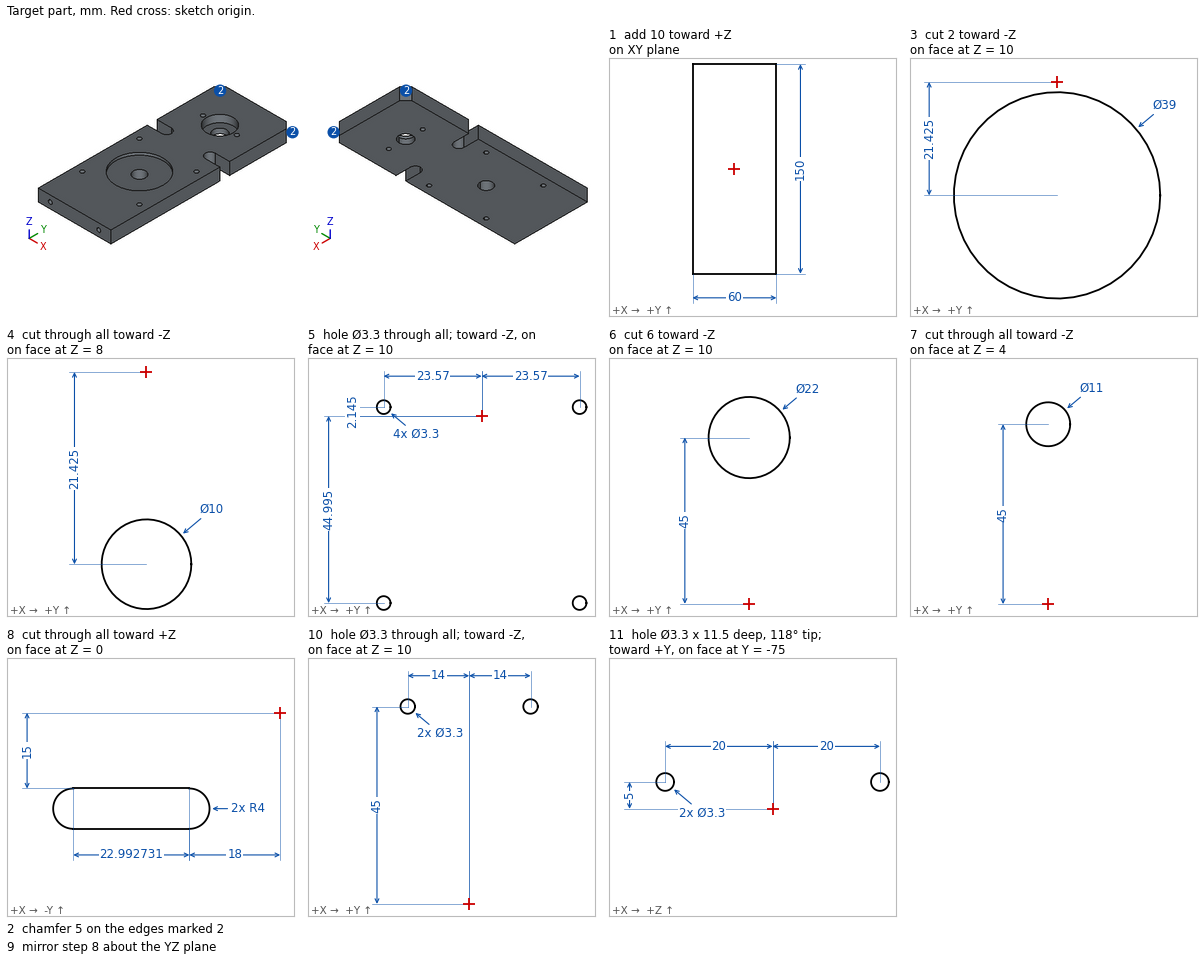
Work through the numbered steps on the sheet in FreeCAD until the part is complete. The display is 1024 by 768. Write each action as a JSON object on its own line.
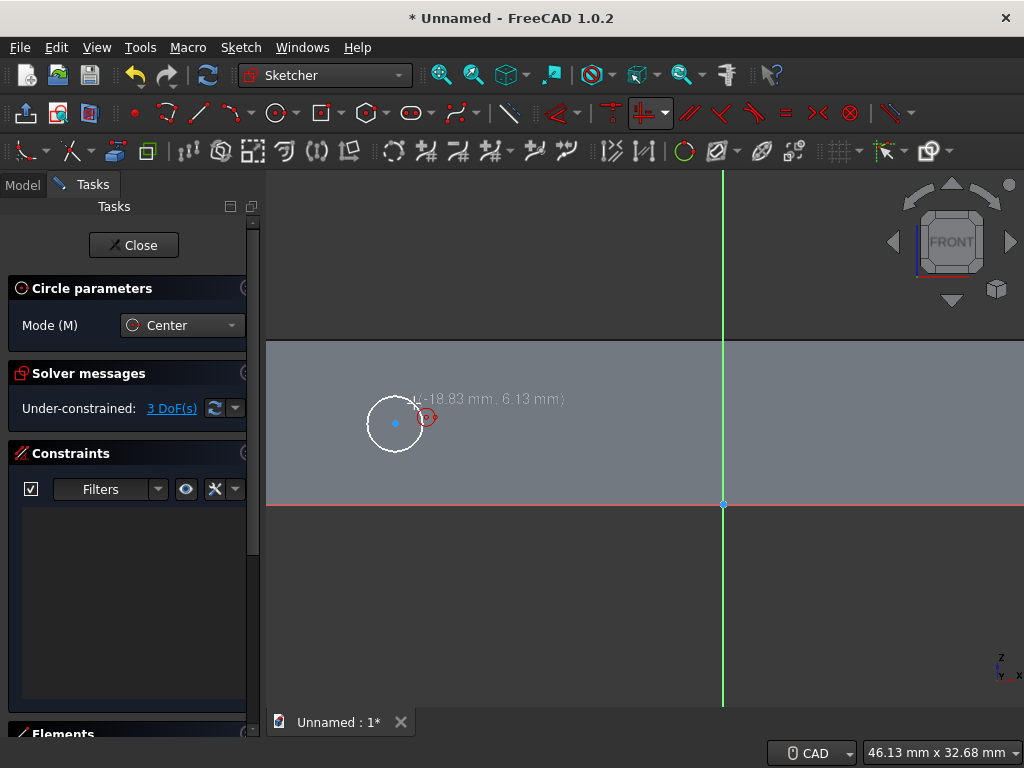
{"action": "scroll", "coordinate": [398, 424], "scroll_direction": "down", "scroll_amount": 3}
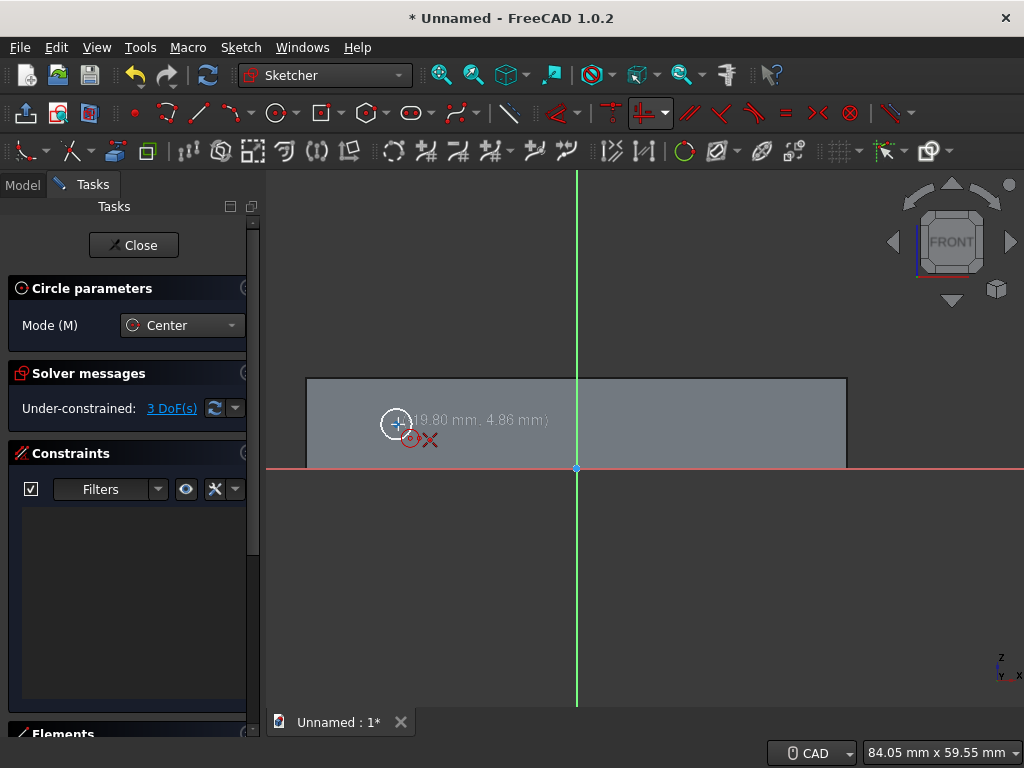
{"action": "scroll", "coordinate": [757, 423], "scroll_direction": "up", "scroll_amount": 3}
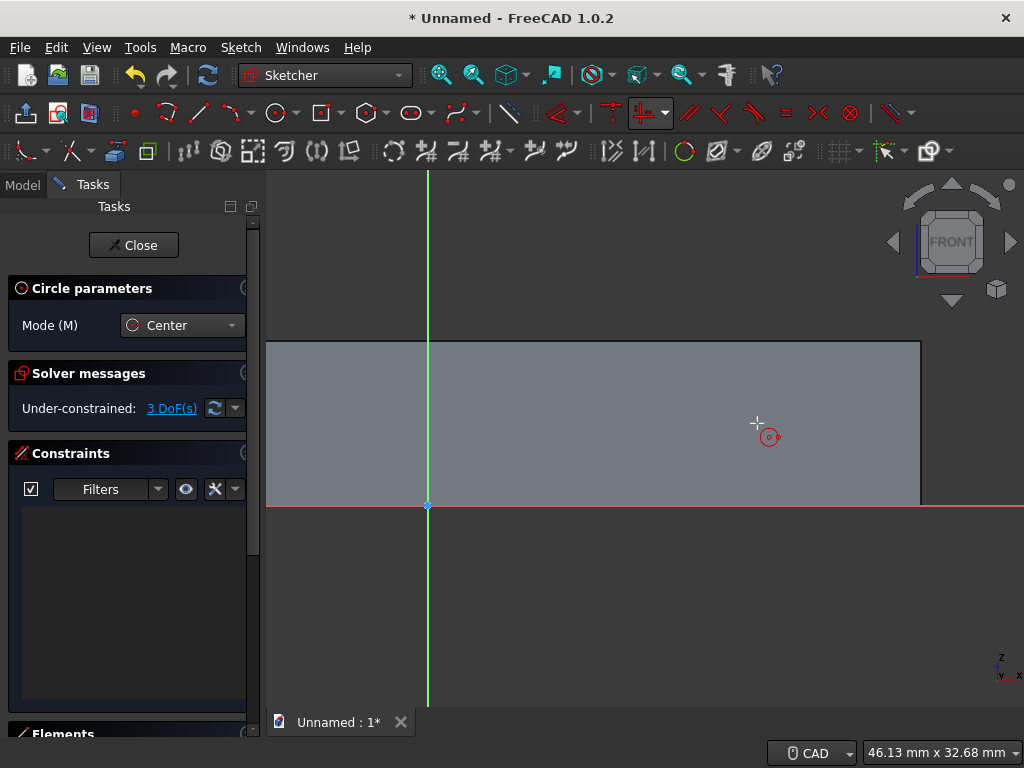
{"action": "left_click", "coordinate": [757, 423]}
{"action": "left_click", "coordinate": [776, 404]}
{"action": "key", "text": "Escape"}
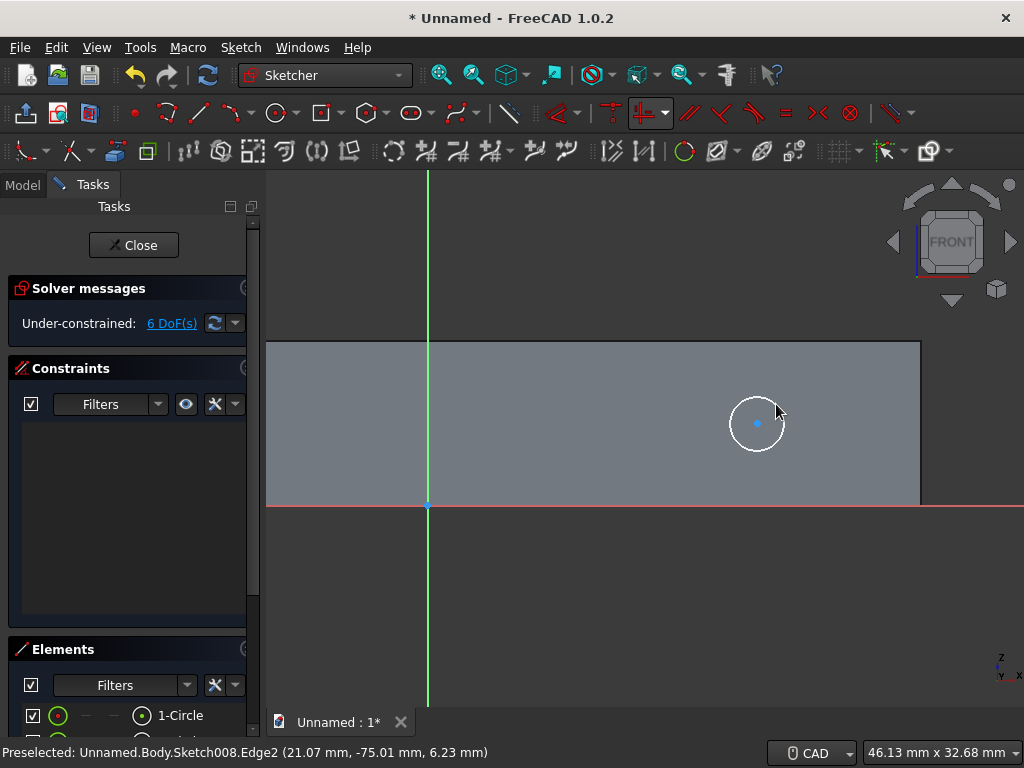
{"action": "scroll", "coordinate": [757, 423], "scroll_direction": "down", "scroll_amount": 3}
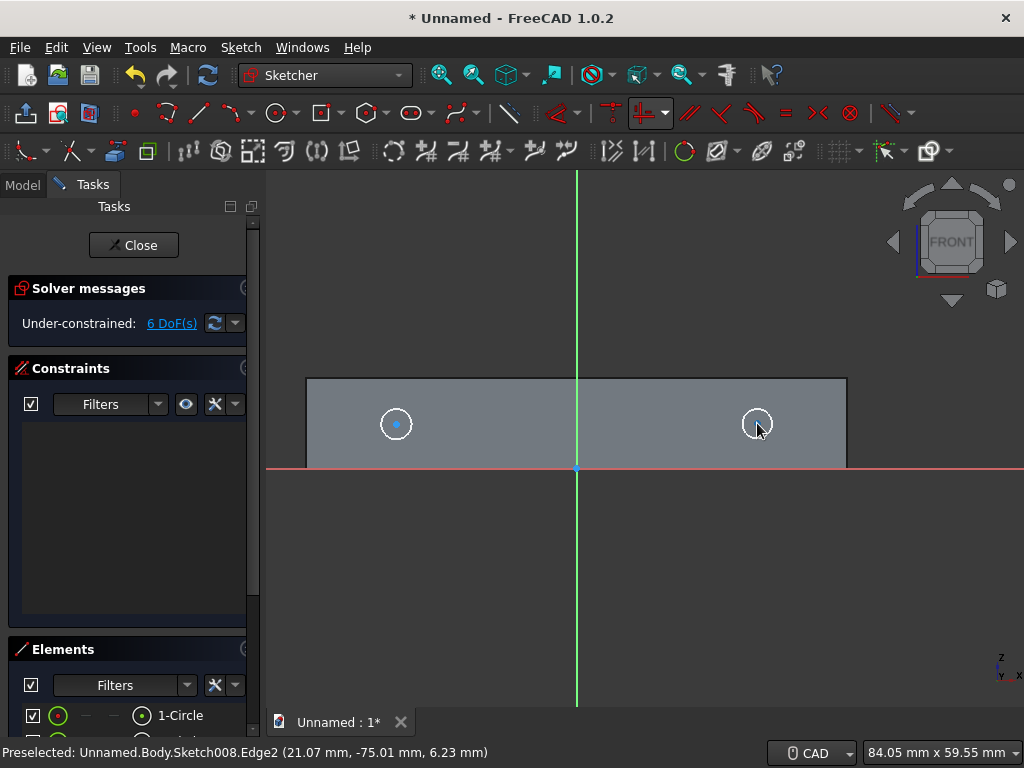
{"action": "left_click", "coordinate": [407, 413]}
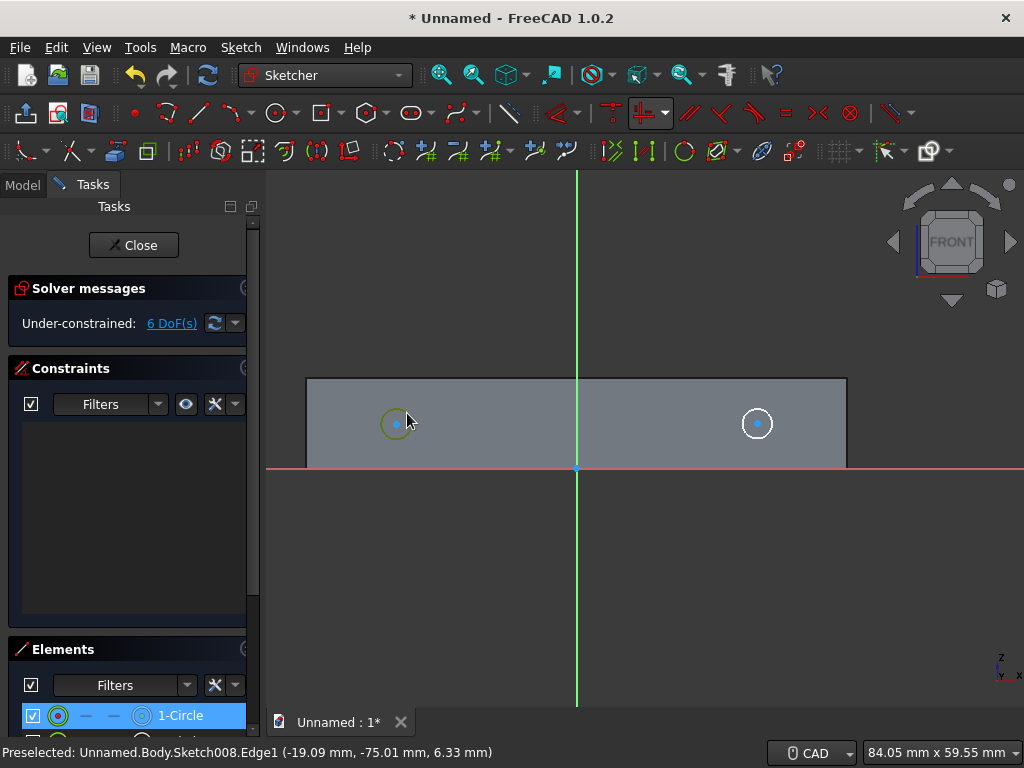
{"action": "left_click", "coordinate": [768, 413]}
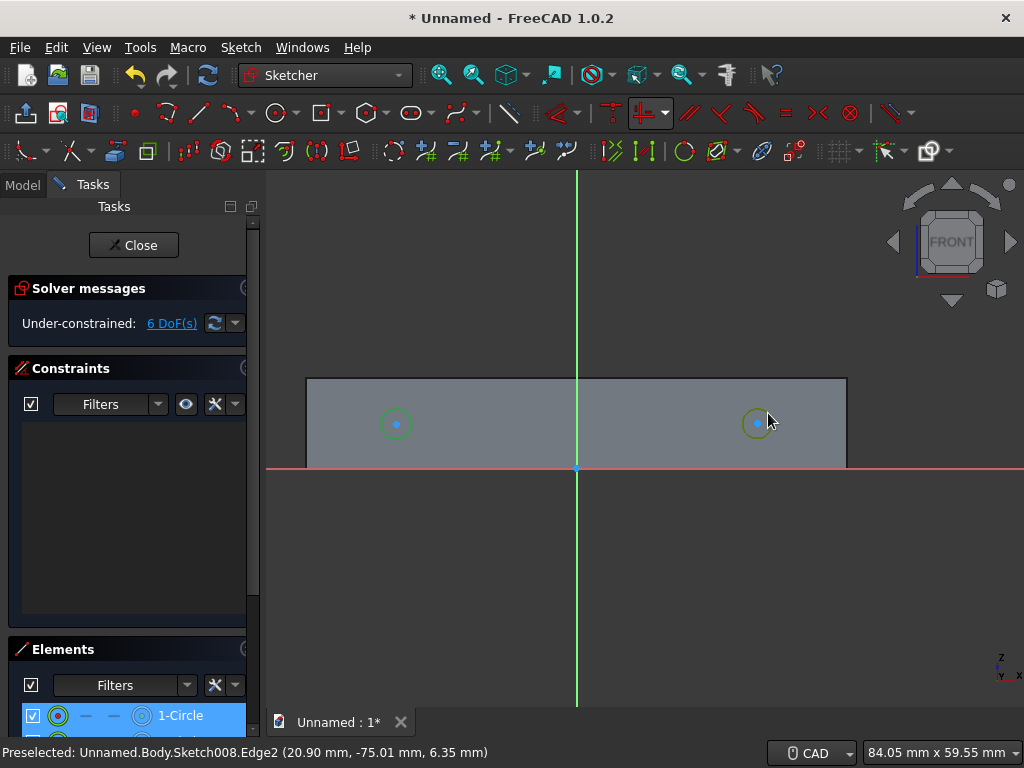
{"action": "left_click", "coordinate": [786, 114]}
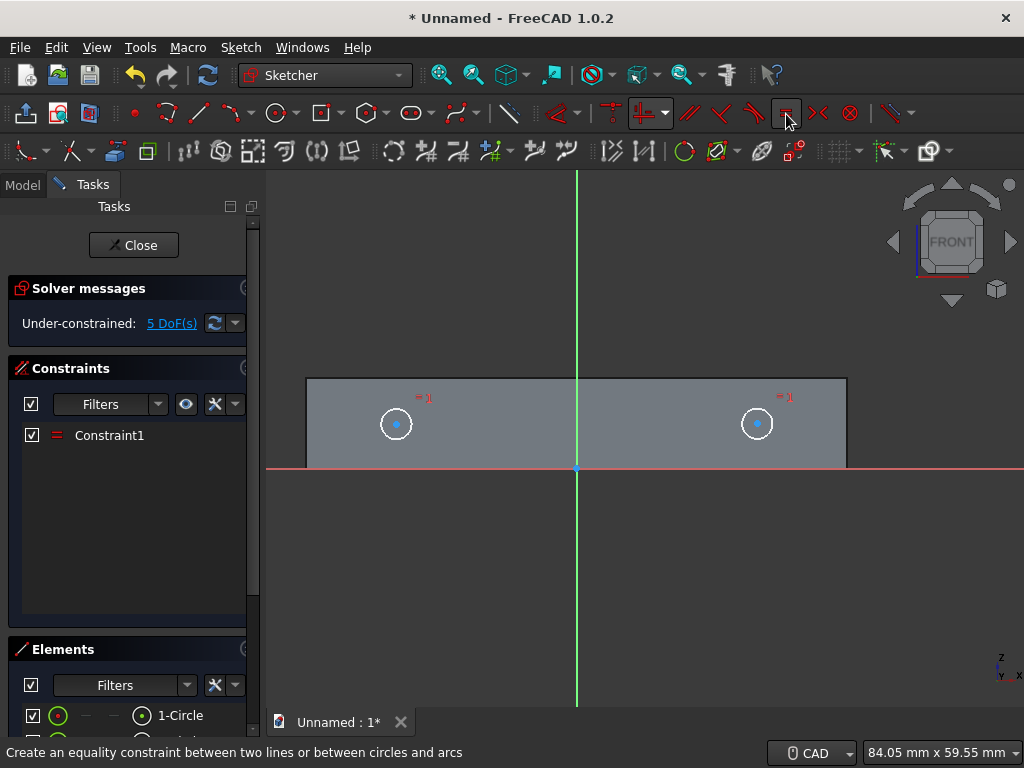
{"action": "left_click", "coordinate": [396, 424]}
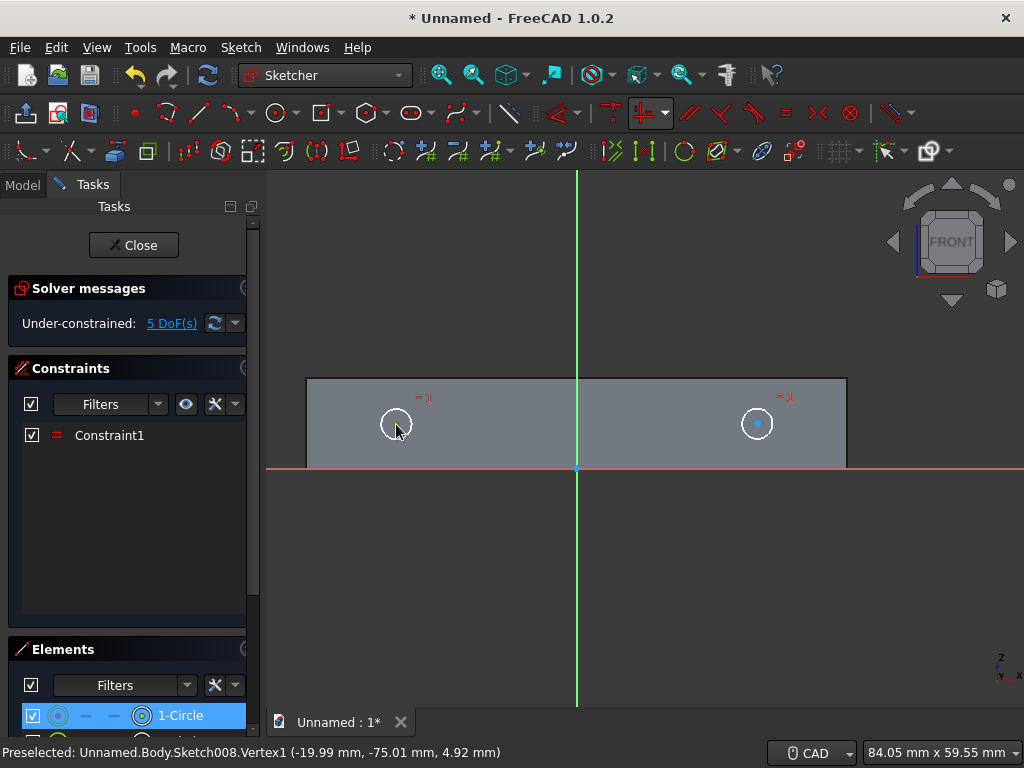
{"action": "left_click", "coordinate": [757, 424]}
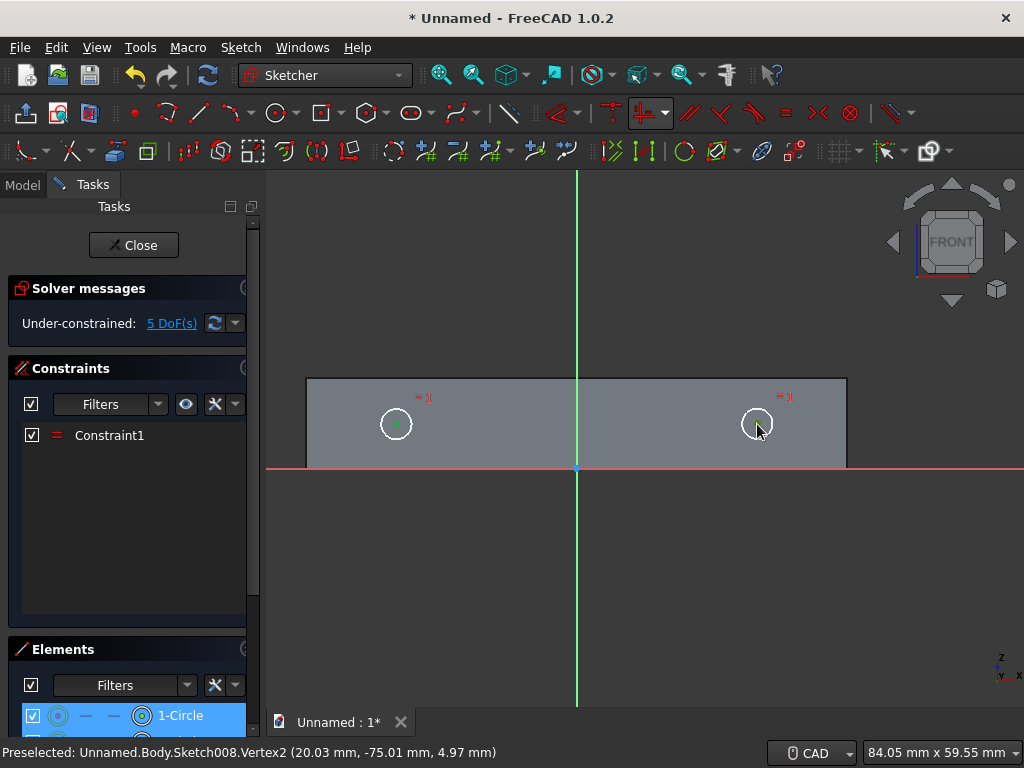
{"action": "key", "text": "h"}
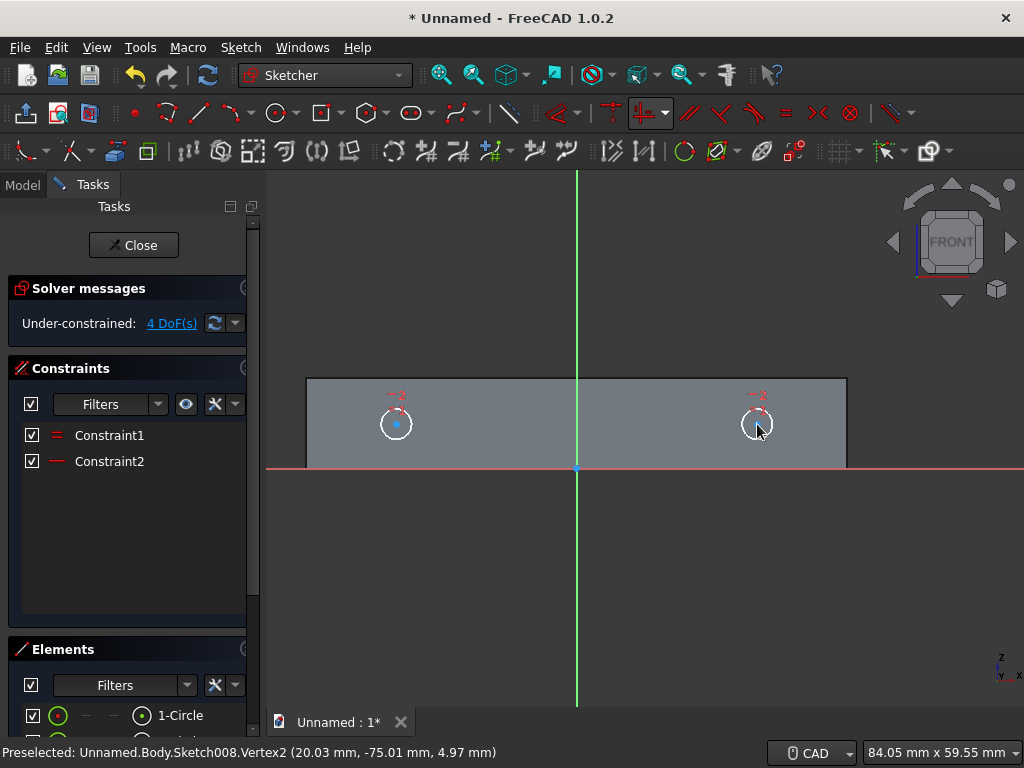
{"action": "left_click", "coordinate": [556, 114]}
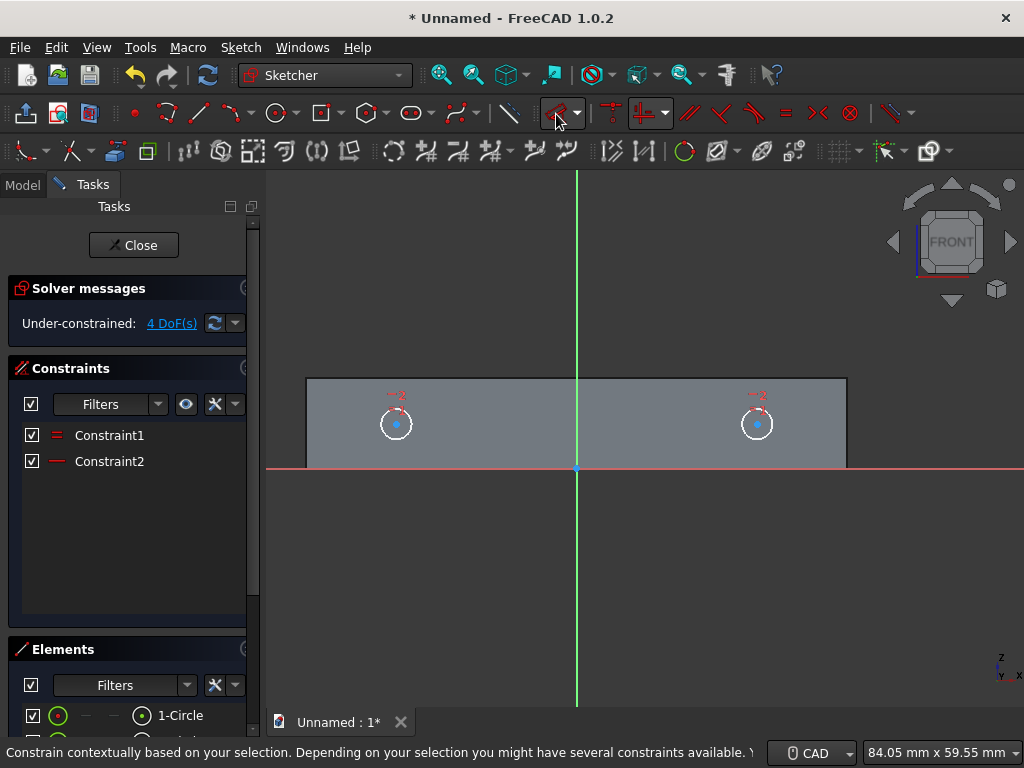
{"action": "scroll", "coordinate": [407, 413], "scroll_direction": "up", "scroll_amount": 2}